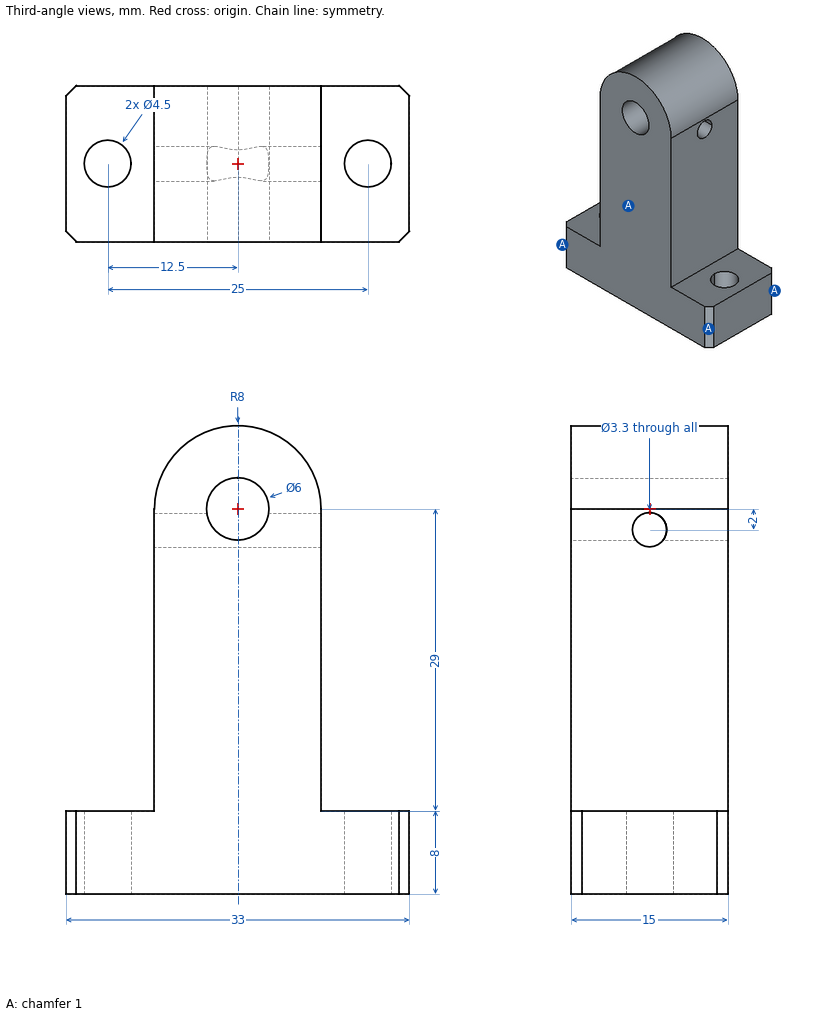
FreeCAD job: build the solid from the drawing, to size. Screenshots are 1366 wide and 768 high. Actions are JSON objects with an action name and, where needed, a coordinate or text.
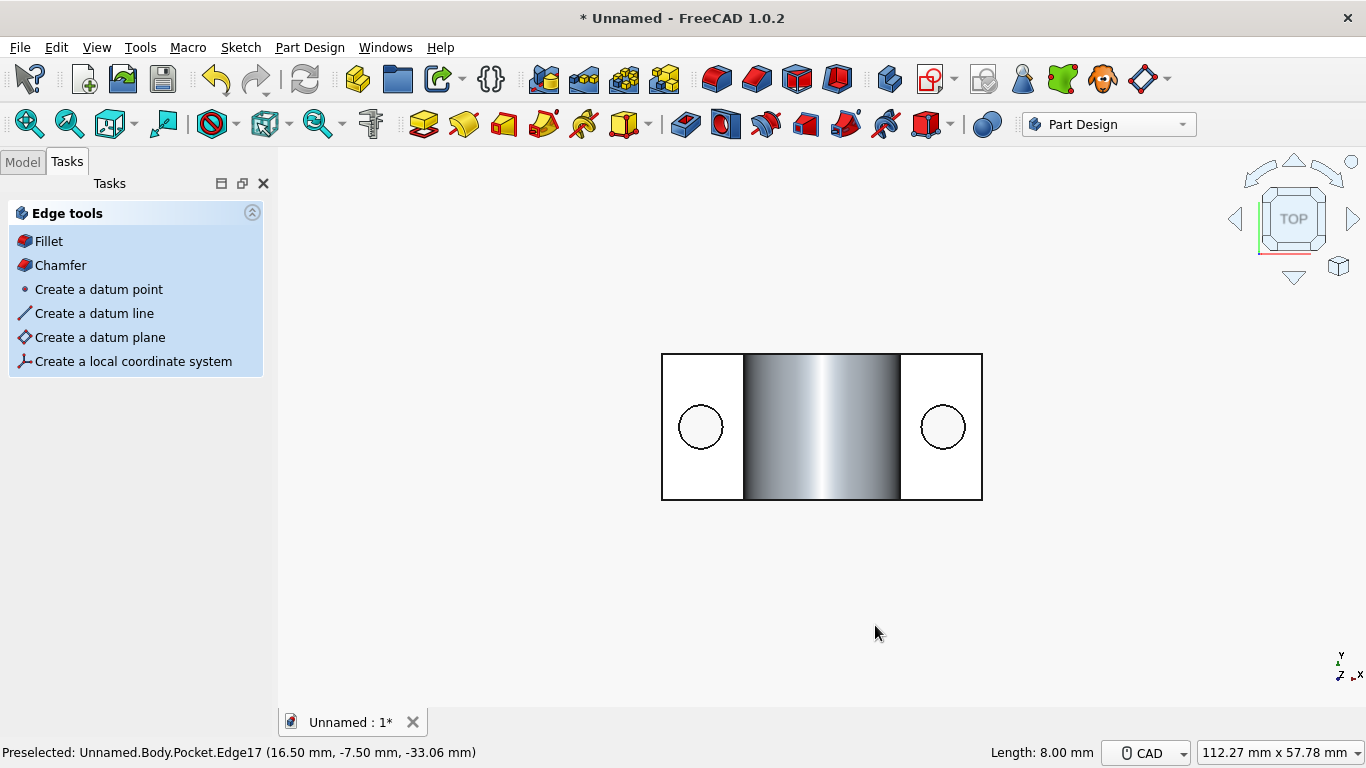
{"action": "key", "text": "1"}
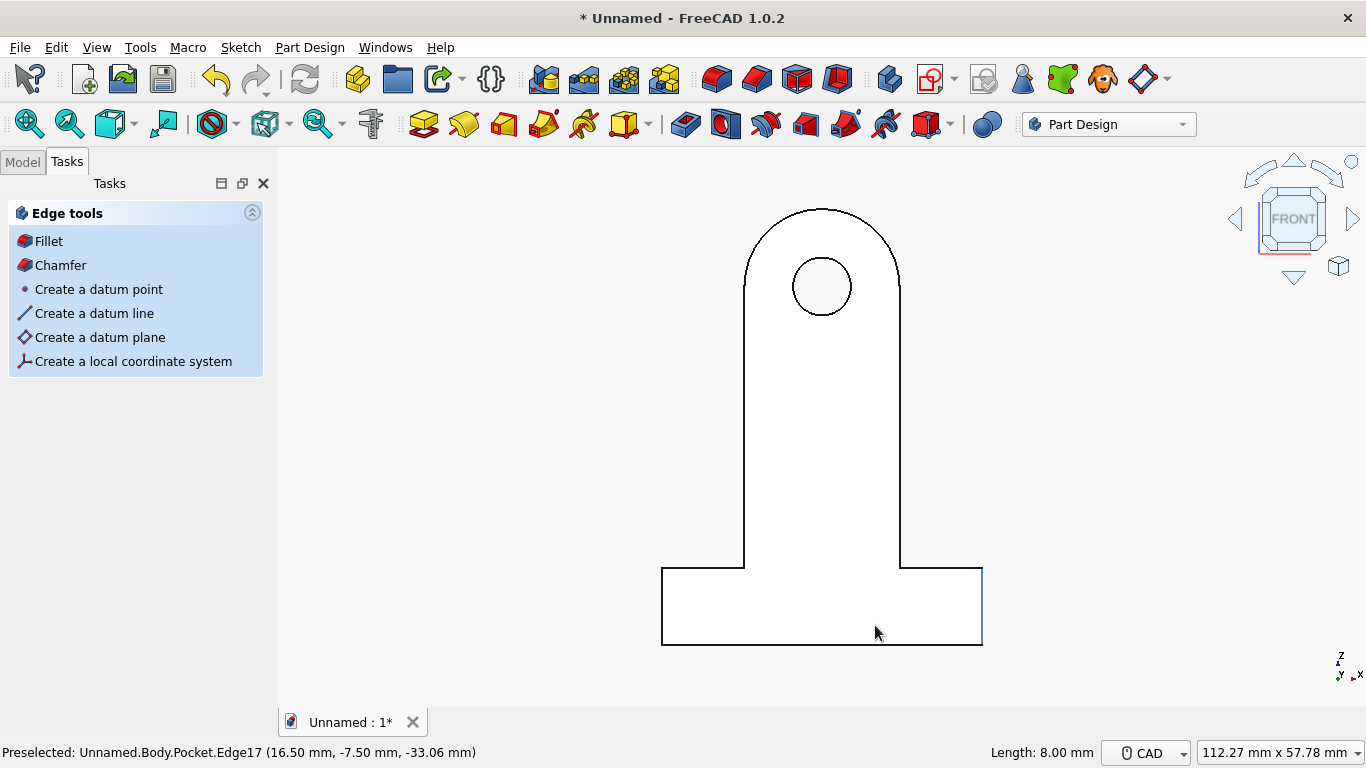
{"action": "left_click", "coordinate": [662, 605], "text": "ctrl"}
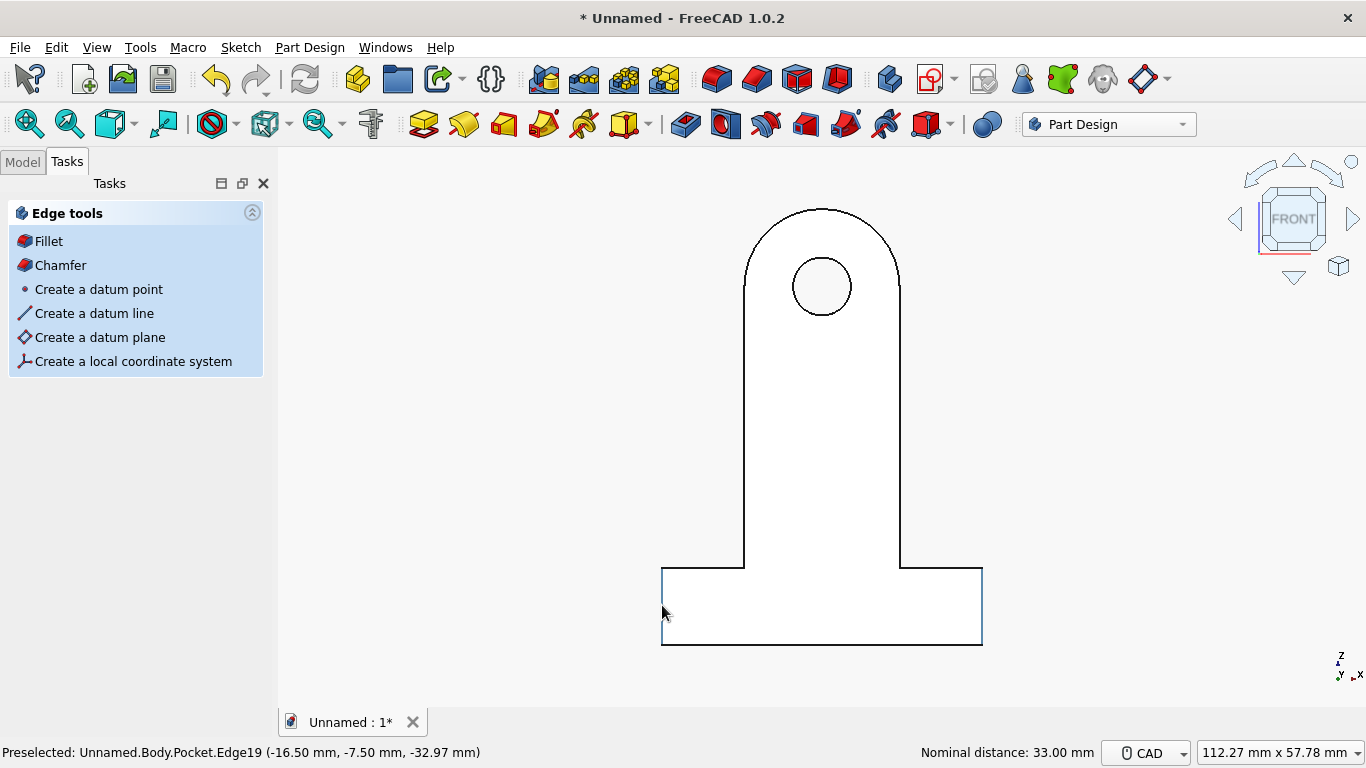
{"action": "key", "text": "3"}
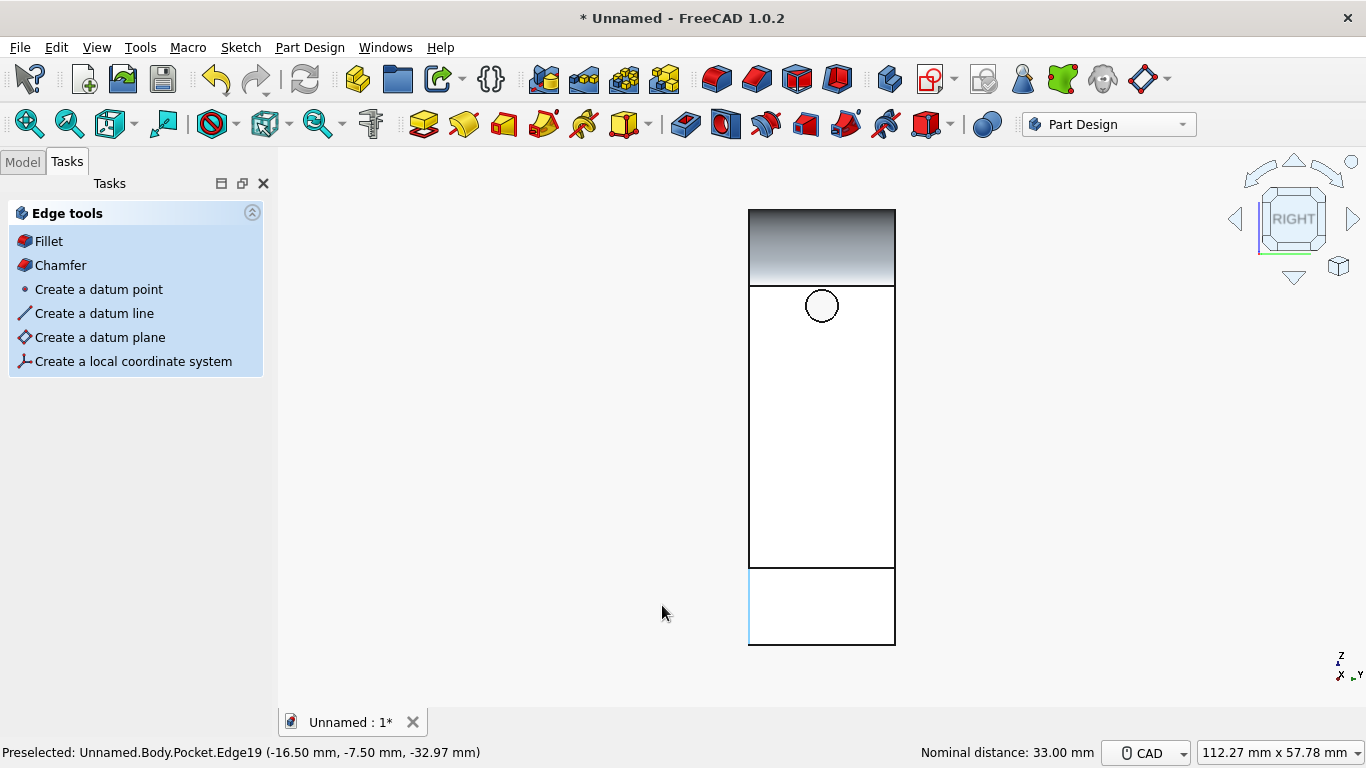
{"action": "left_click", "coordinate": [895, 605], "text": "ctrl"}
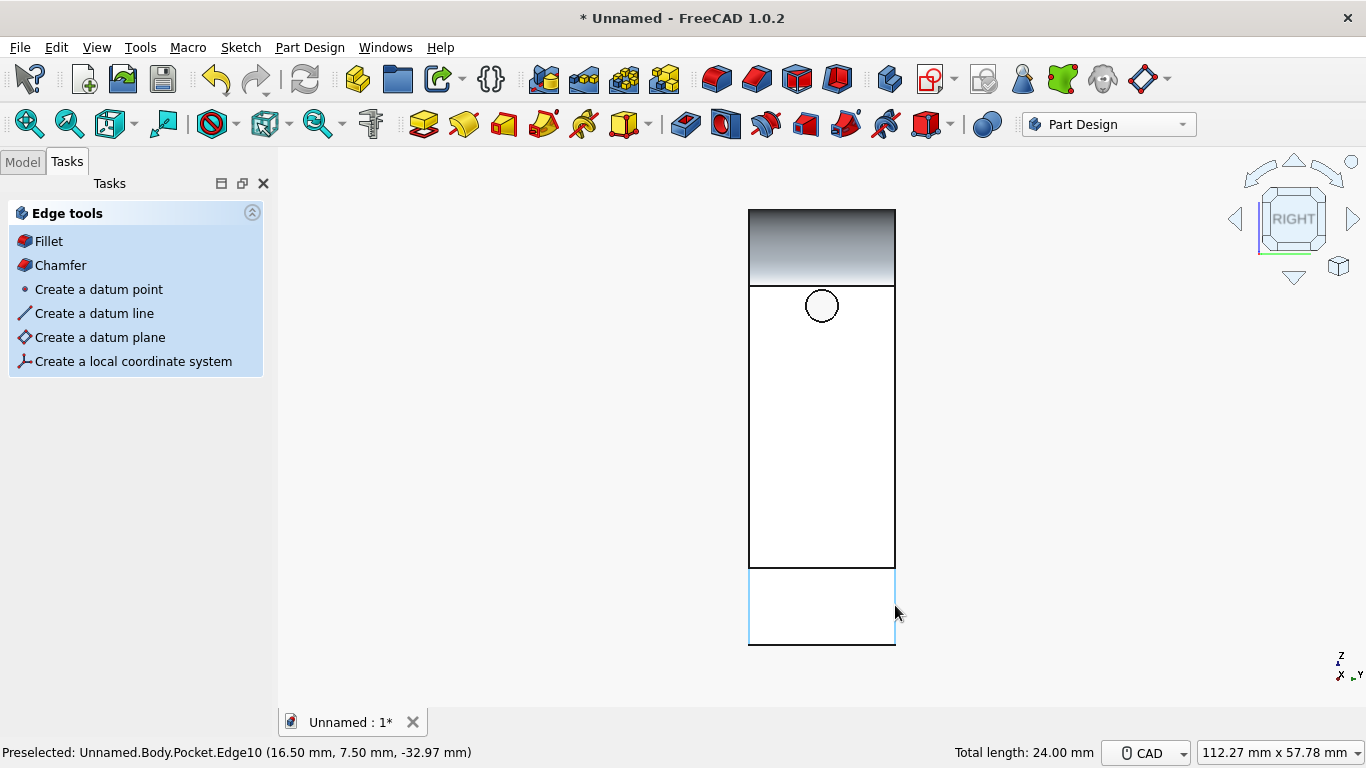
{"action": "key", "text": "5"}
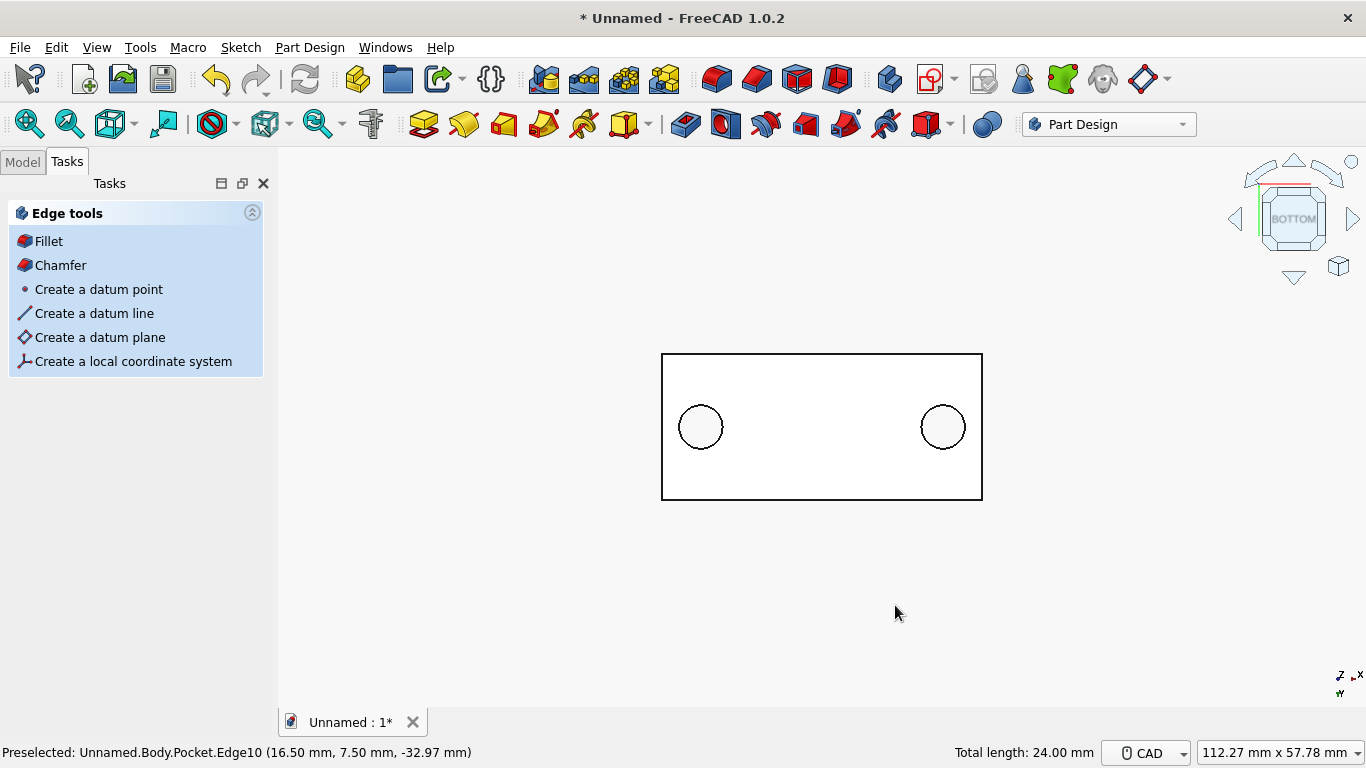
{"action": "left_click", "coordinate": [30, 124]}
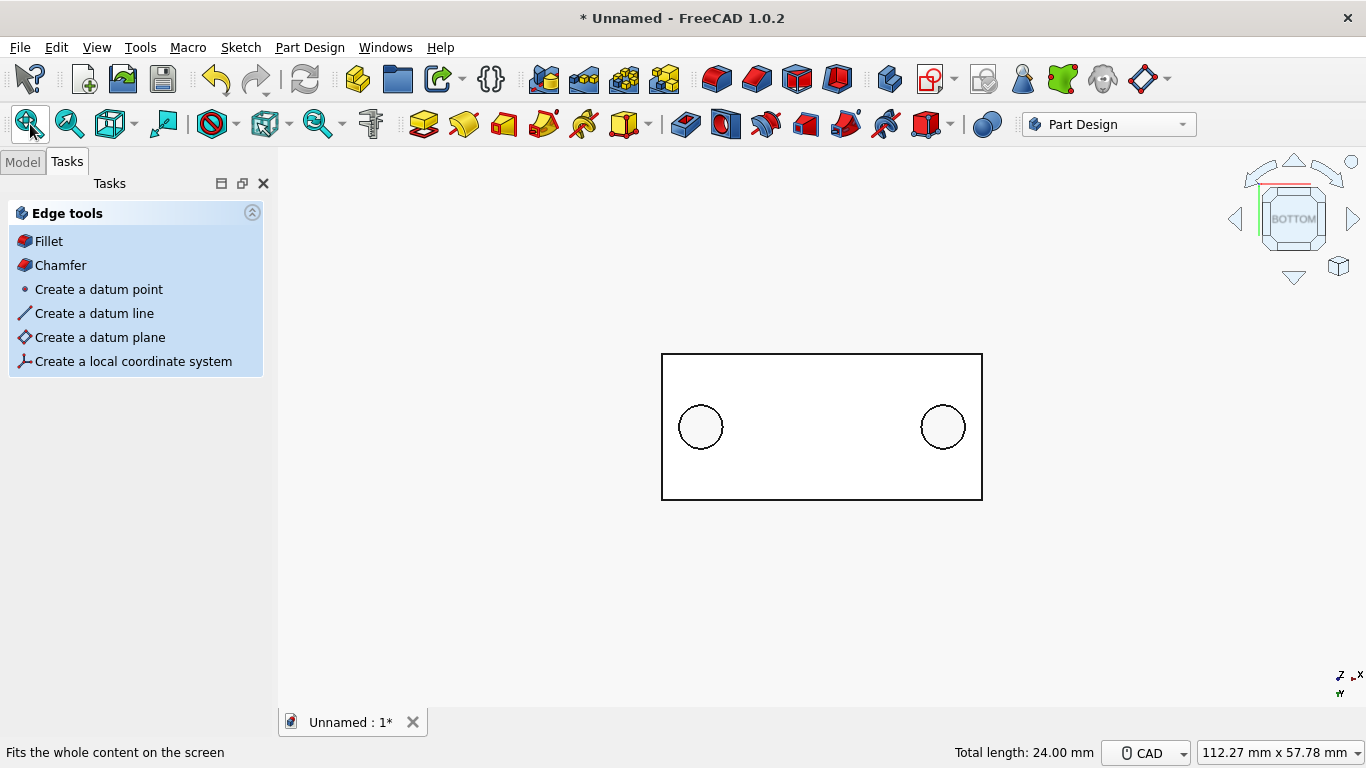
{"action": "key", "text": "4"}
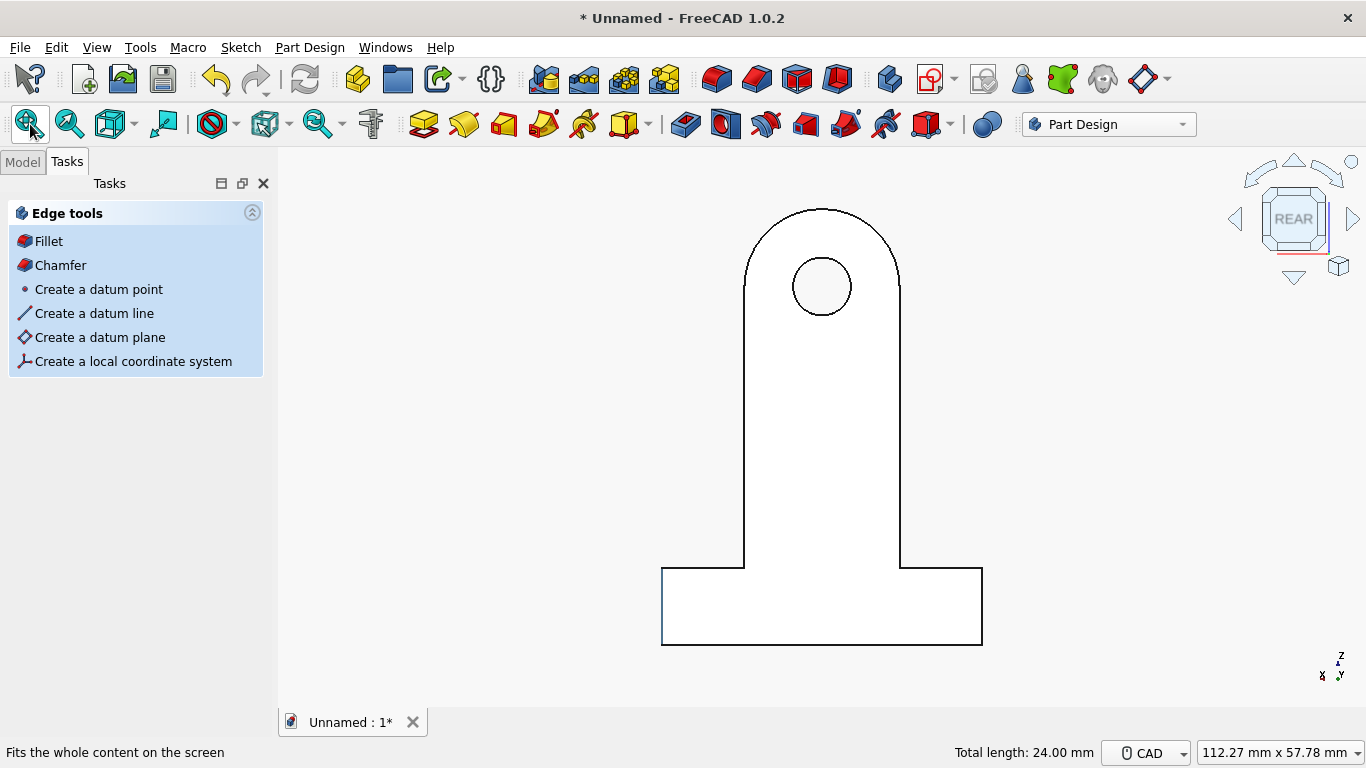
{"action": "left_click", "coordinate": [982, 605], "text": "ctrl"}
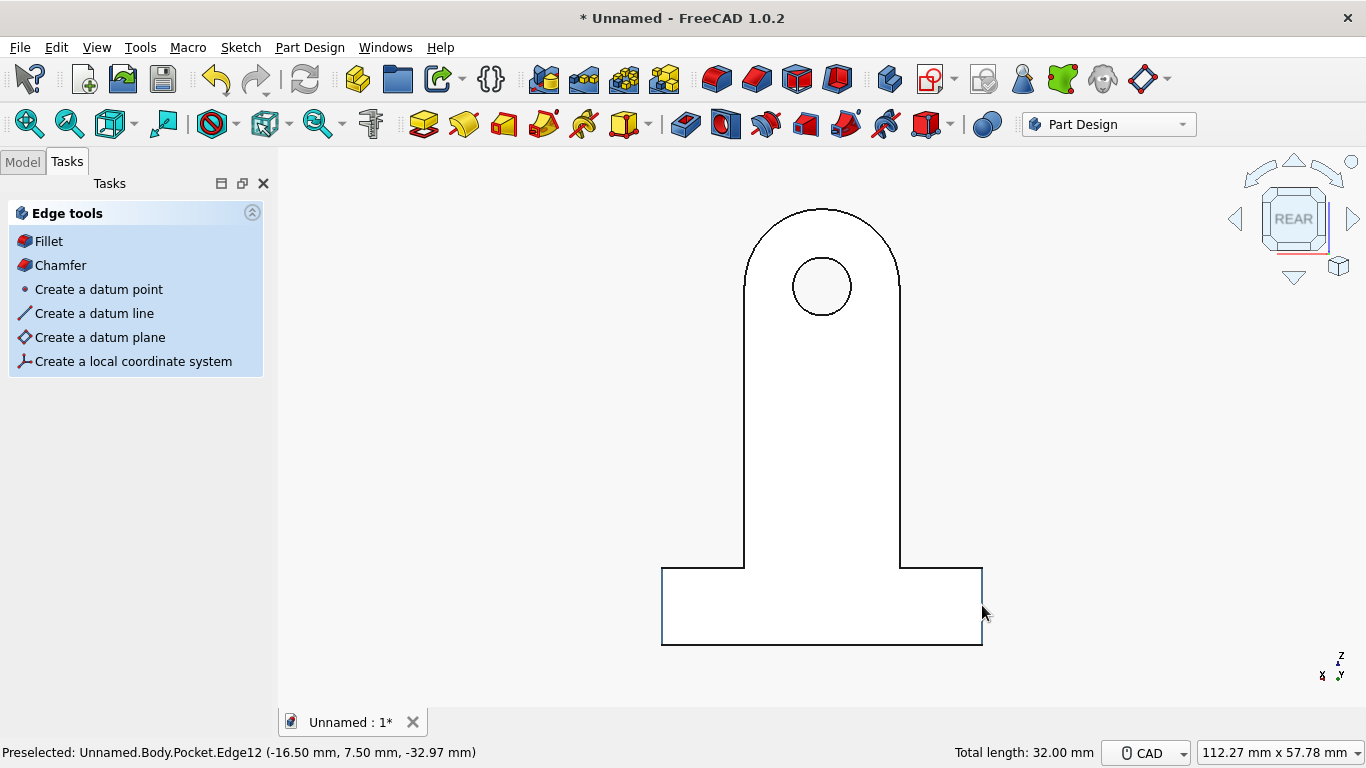
{"action": "left_click", "coordinate": [758, 80]}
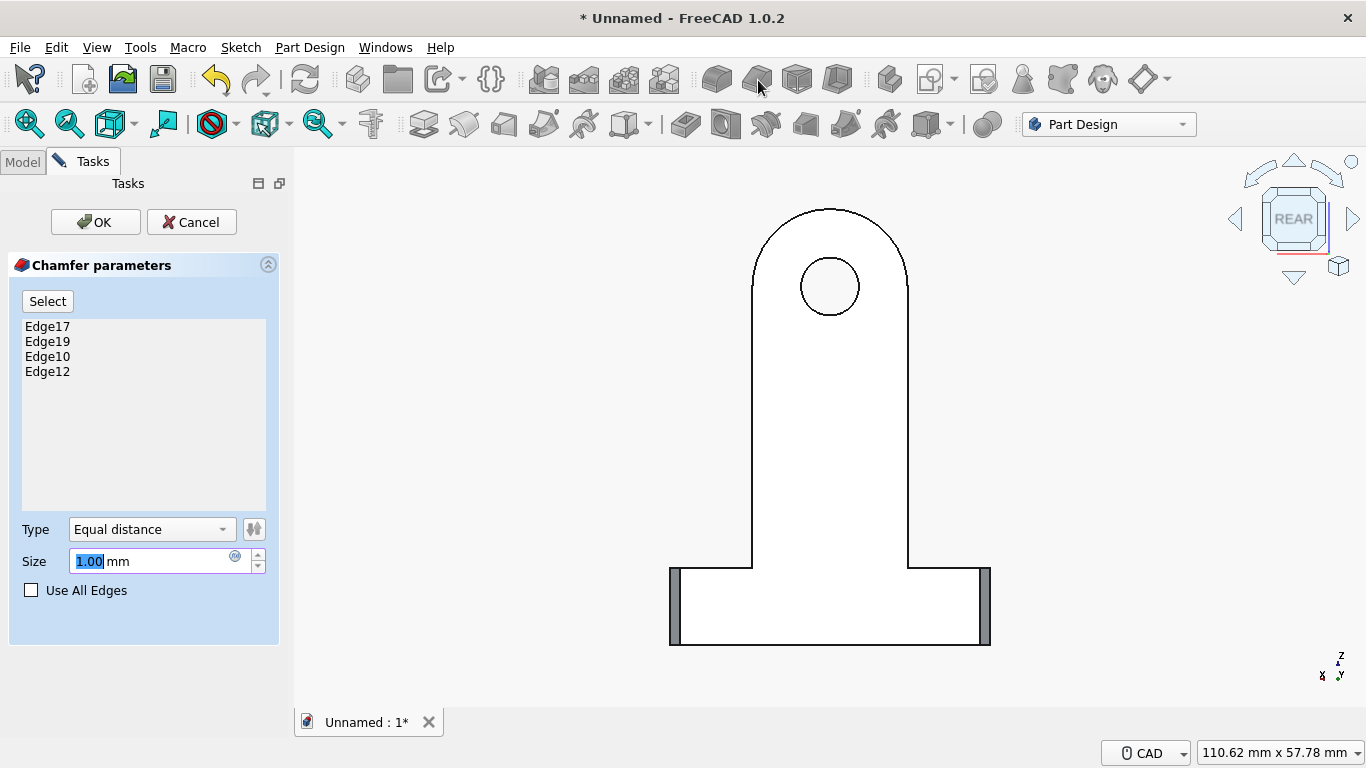
{"action": "type", "text": "1"}
{"action": "key", "text": "Tab"}